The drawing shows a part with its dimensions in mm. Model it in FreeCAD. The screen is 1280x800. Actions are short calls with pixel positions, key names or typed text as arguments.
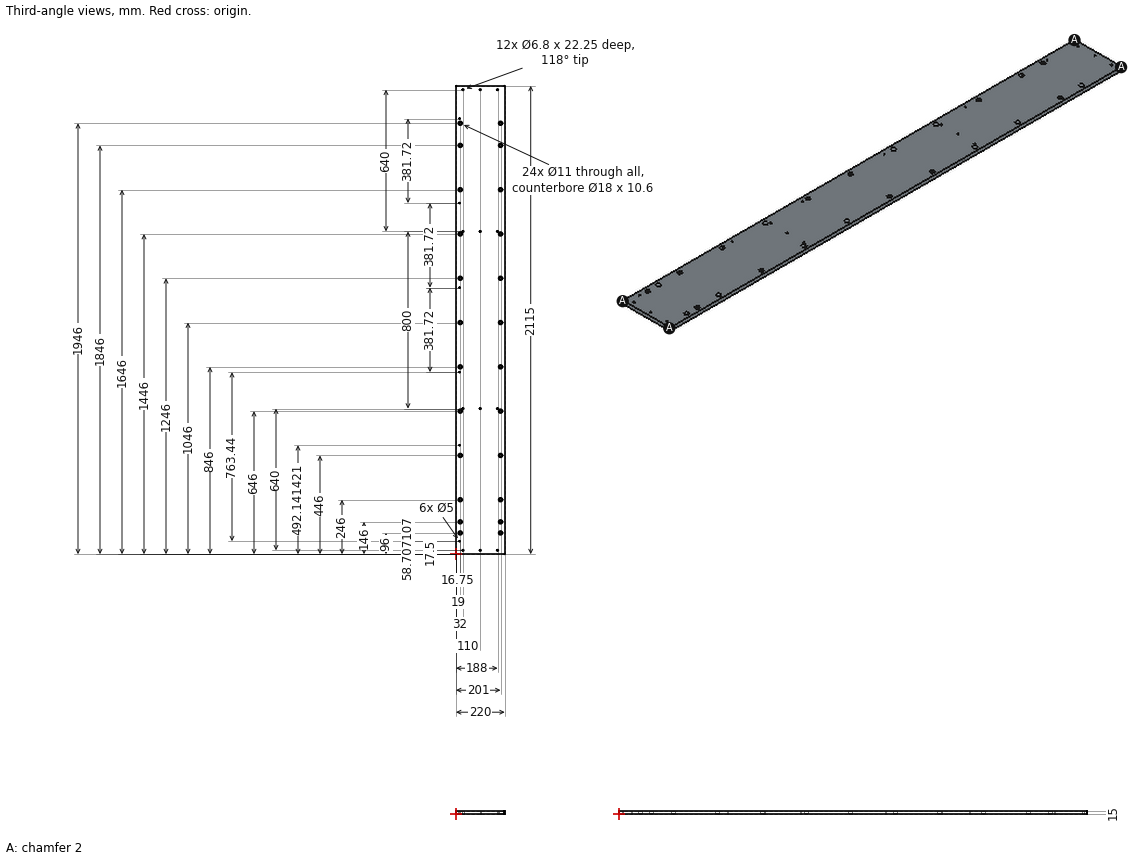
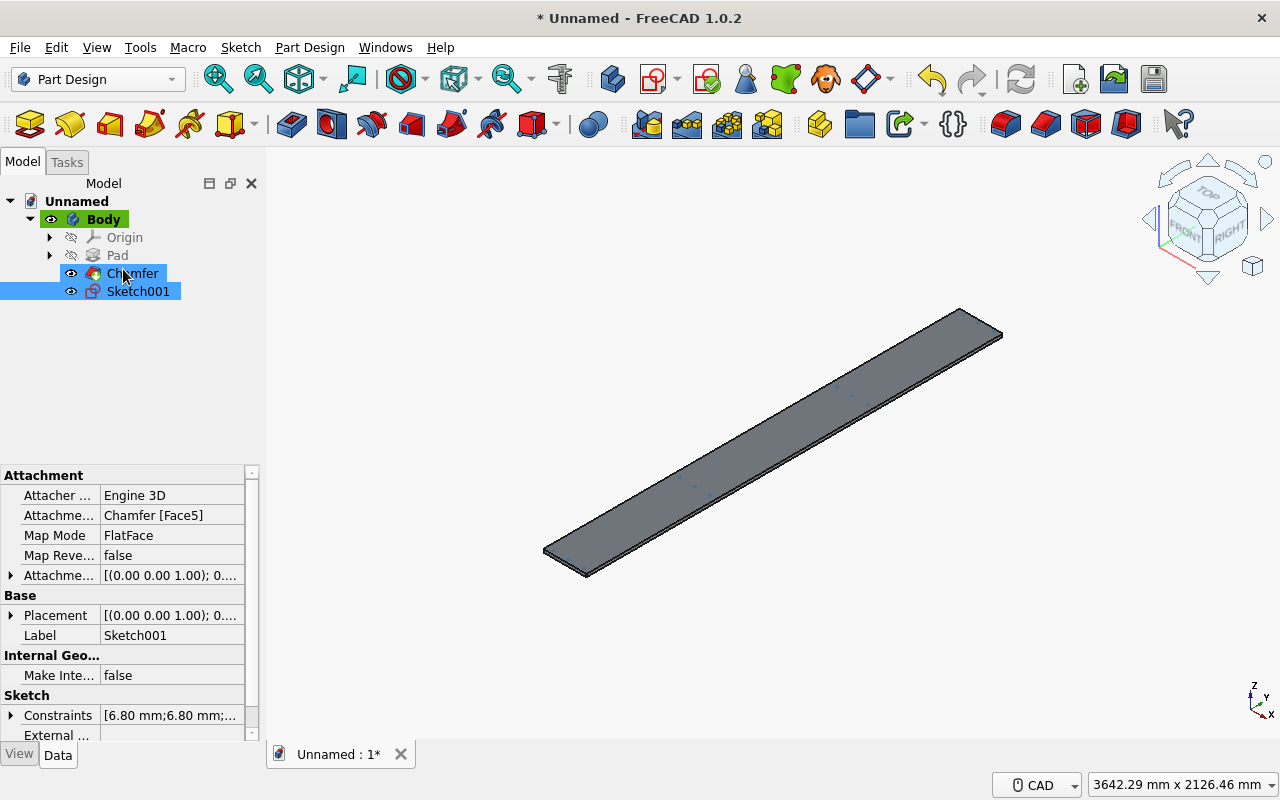
click(332, 124)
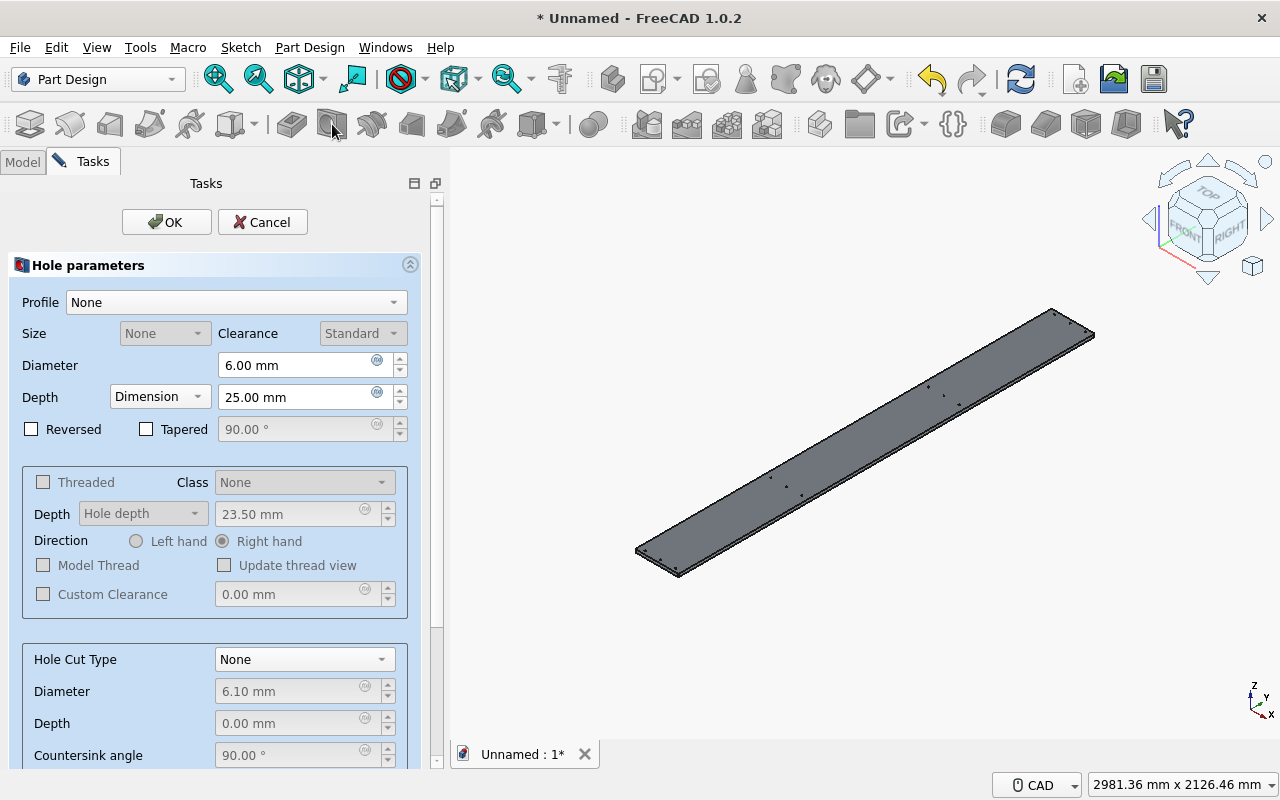
triple_click(305, 365)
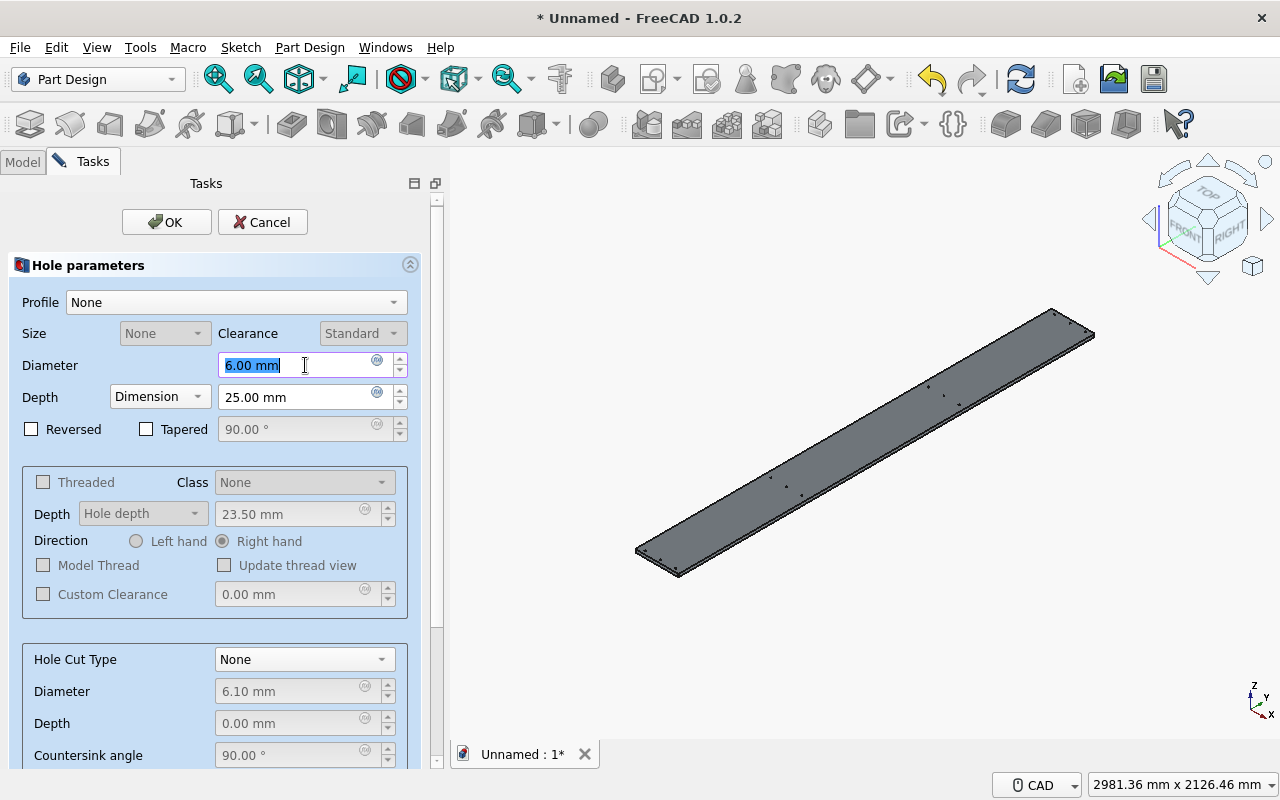
text(6.8)
key(Tab)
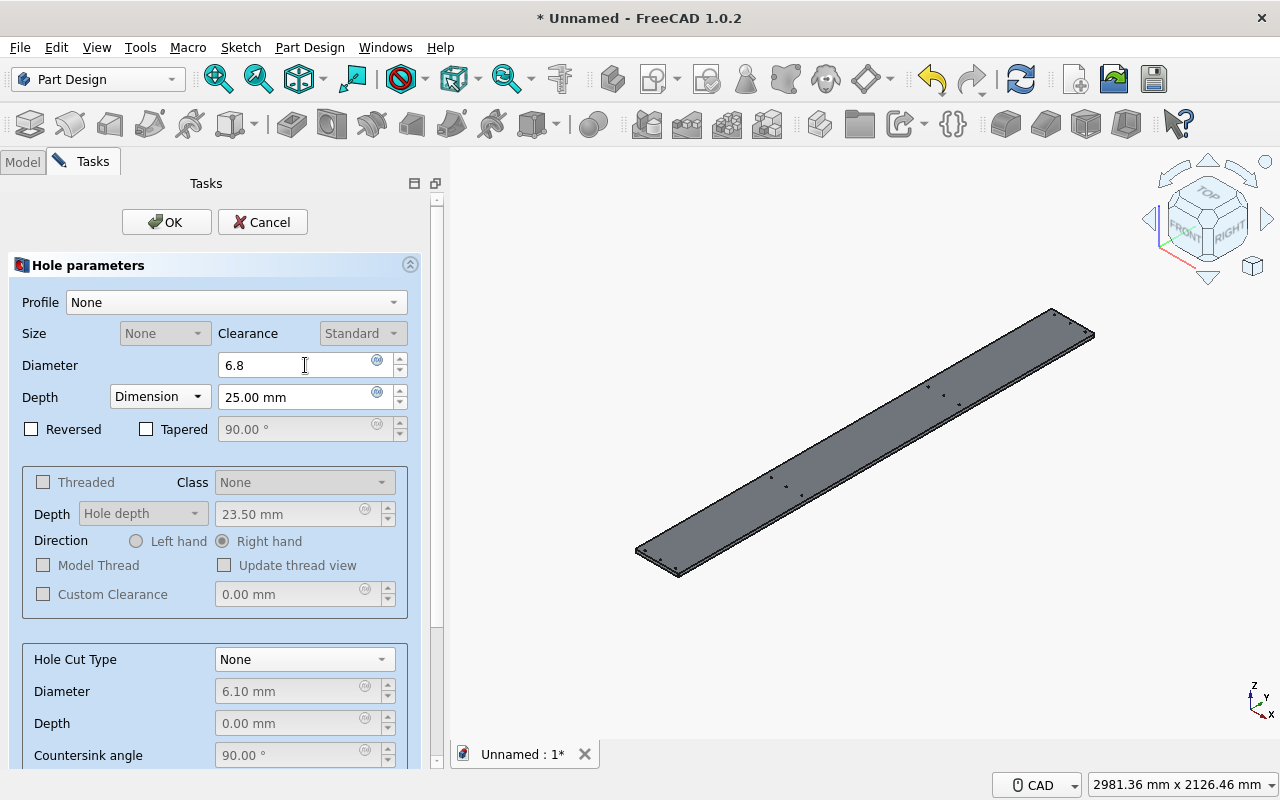
triple_click(305, 397)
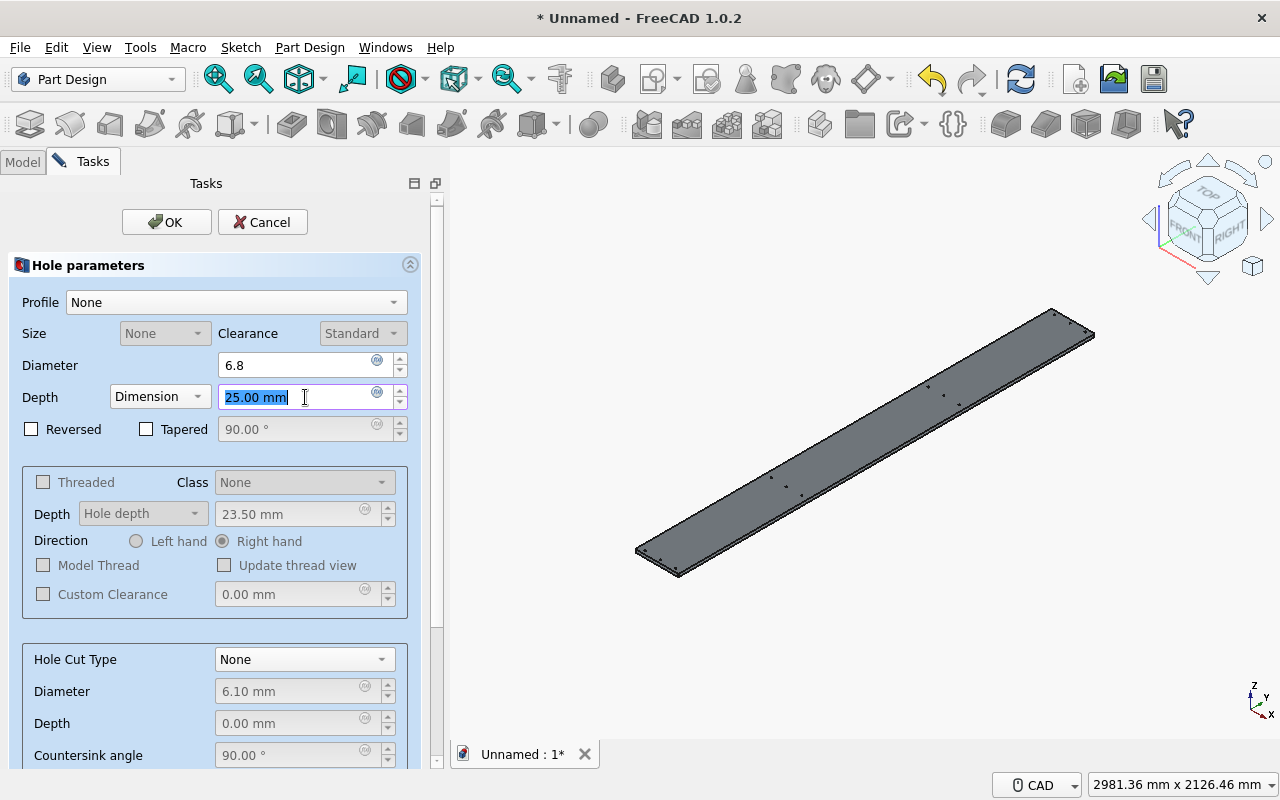
text(22.25)
key(Tab)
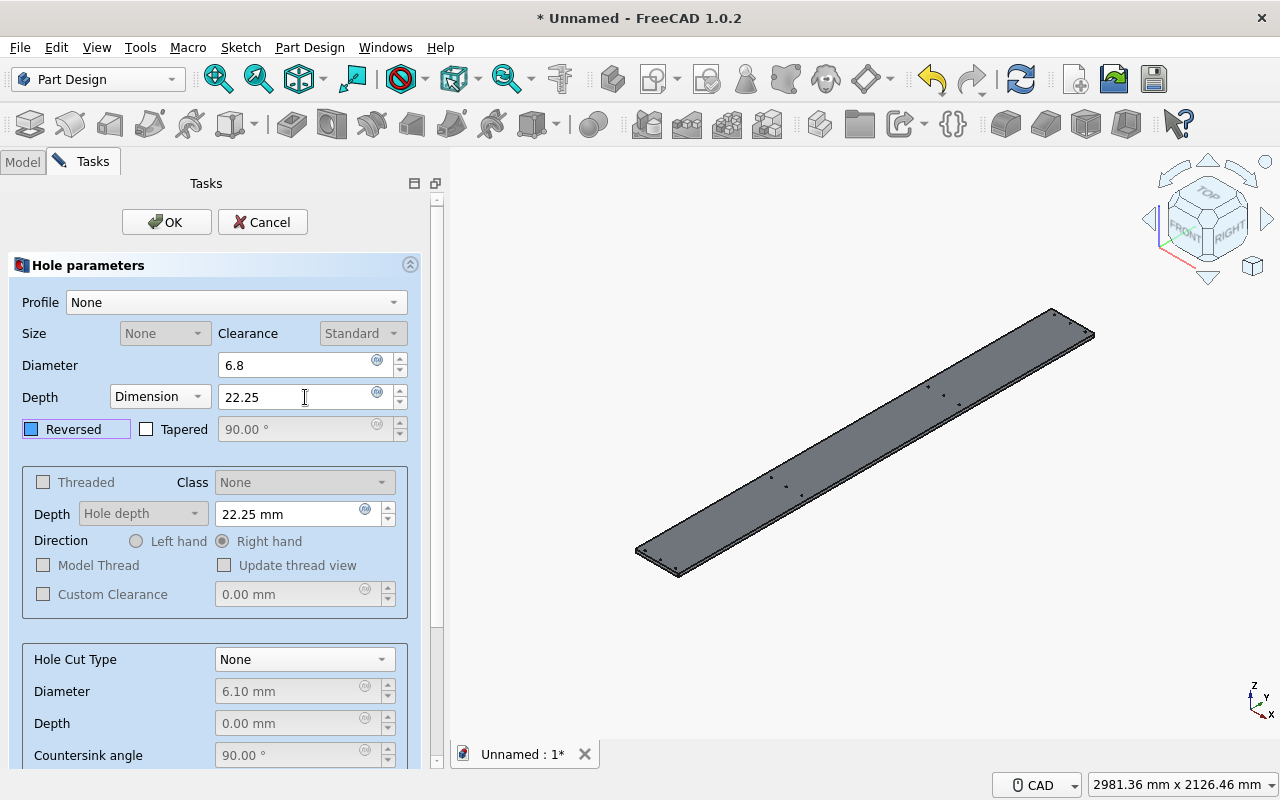
click(167, 222)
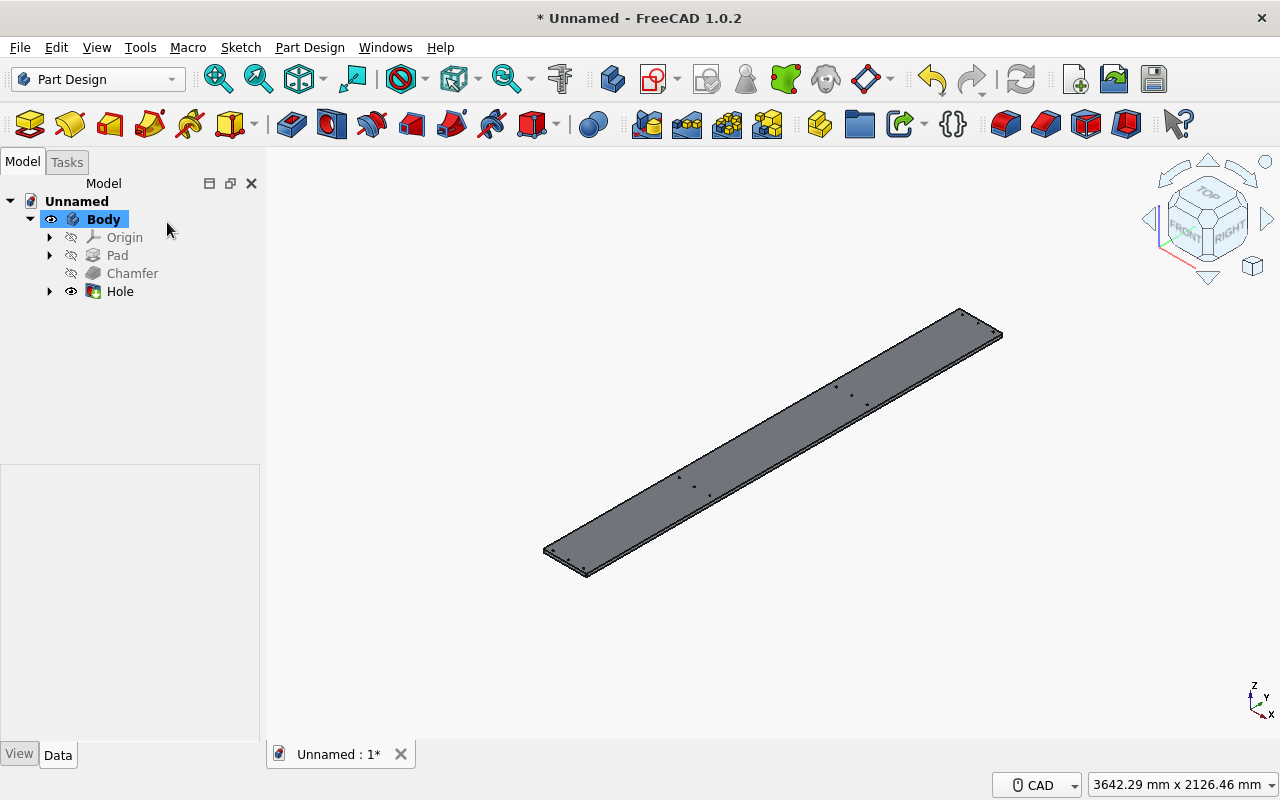
click(951, 337)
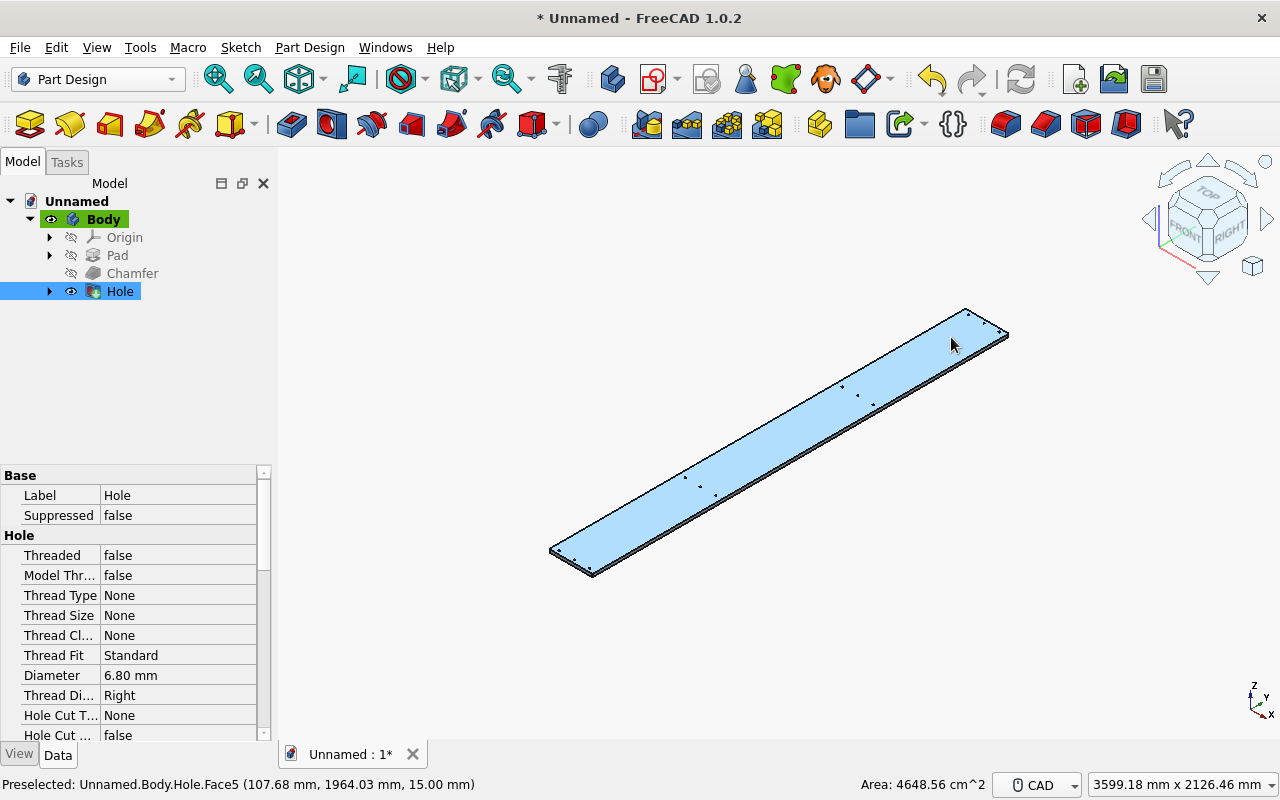
click(654, 80)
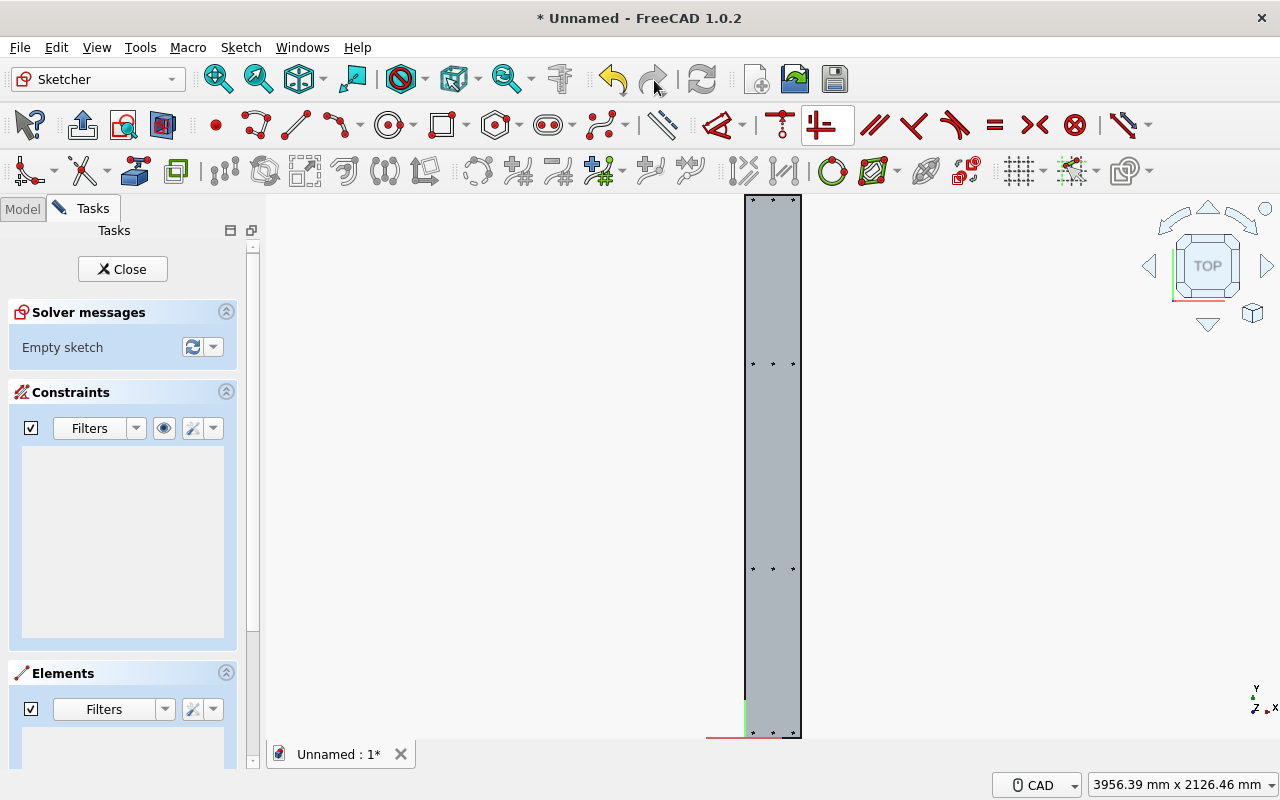
scroll(569, 424, down, 2)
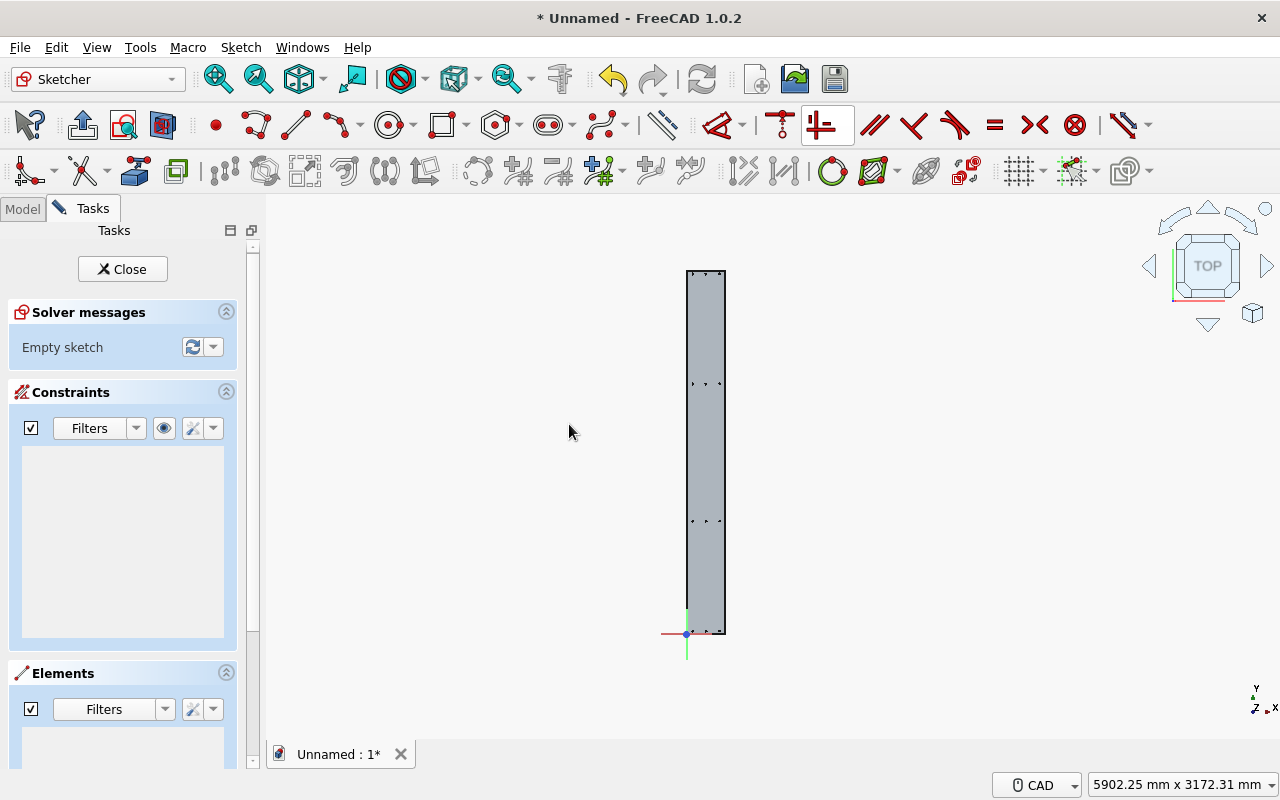
click(390, 126)